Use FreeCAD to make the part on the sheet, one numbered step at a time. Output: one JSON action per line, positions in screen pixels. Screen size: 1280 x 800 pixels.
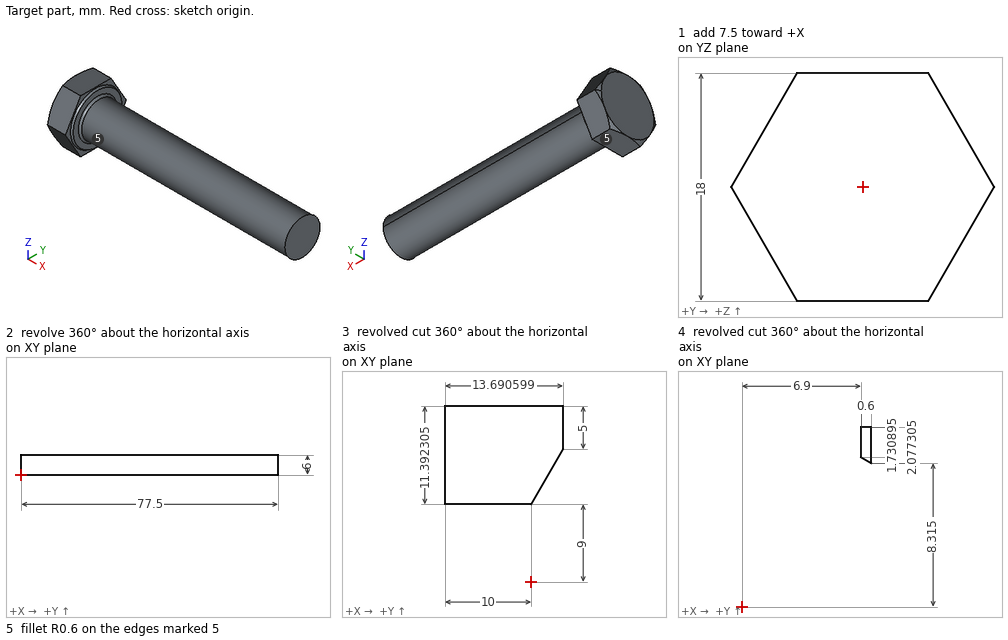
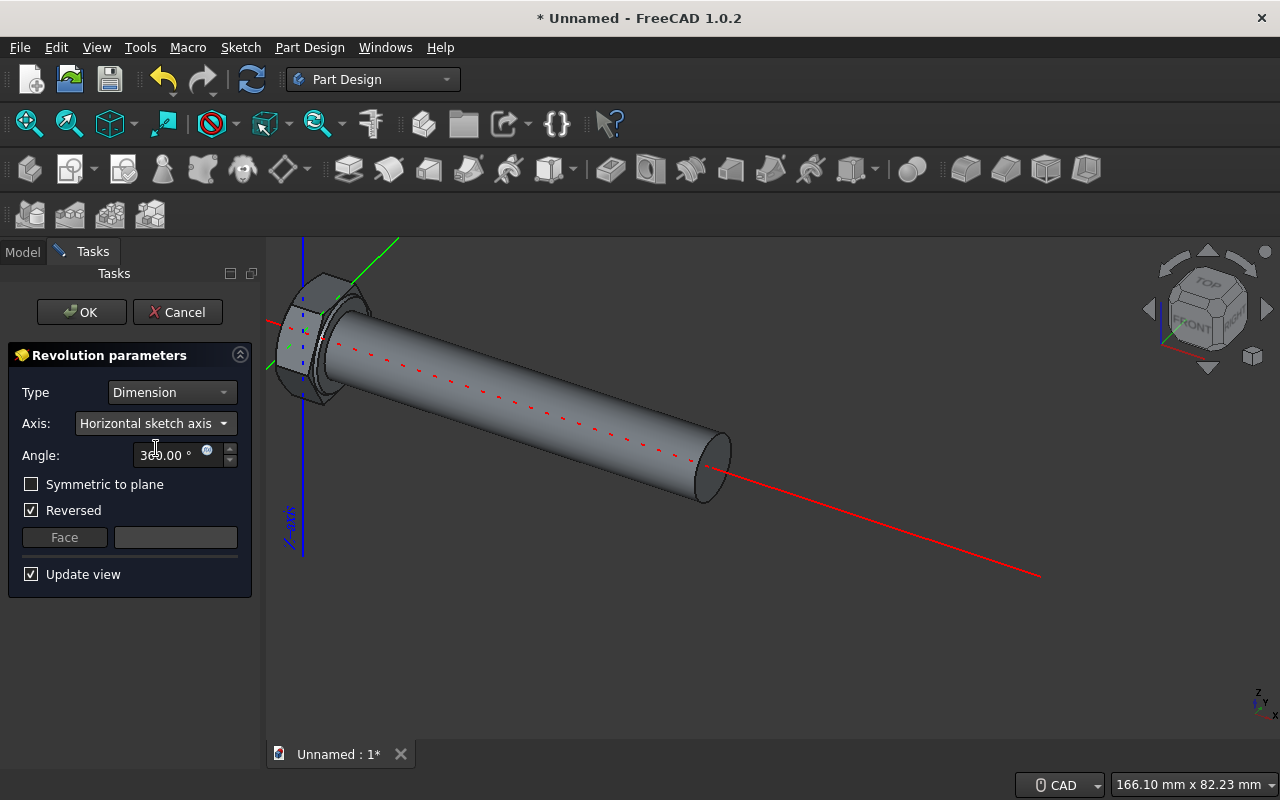
{"action": "left_click", "coordinate": [82, 312]}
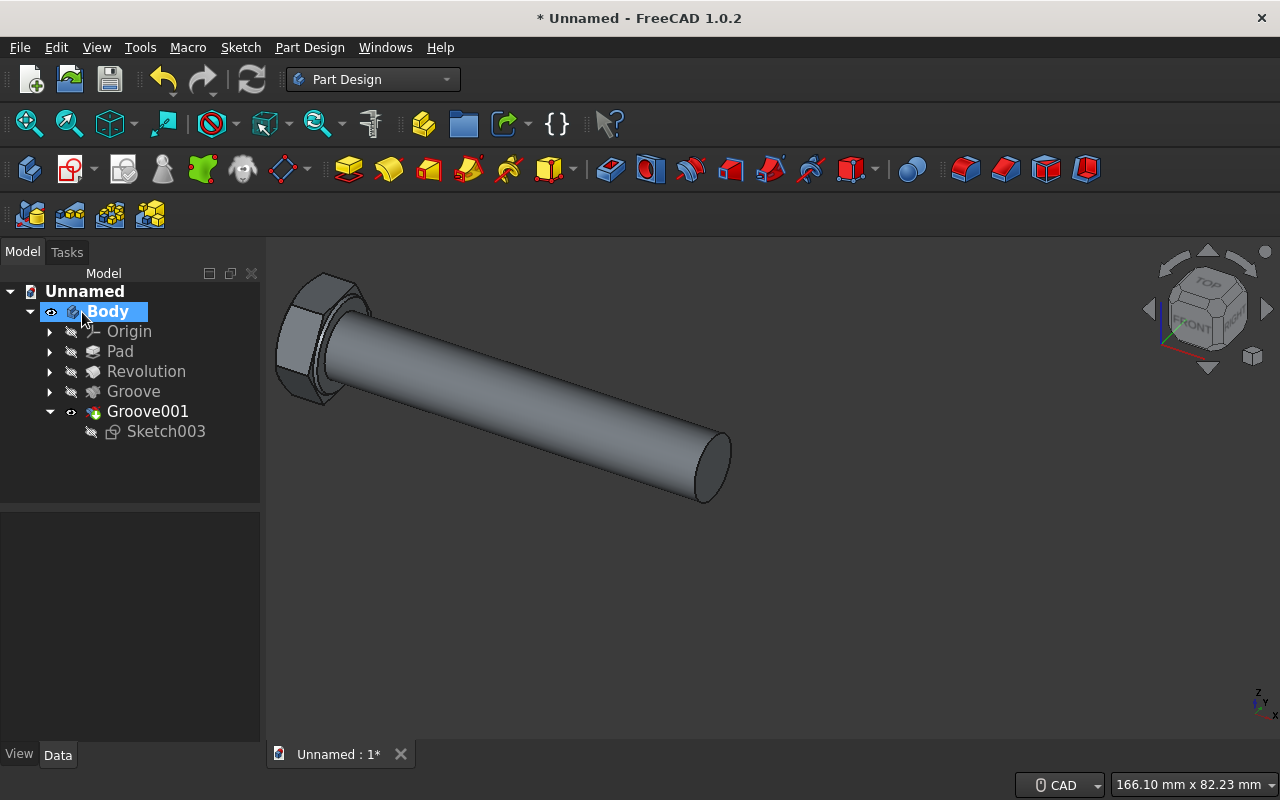
{"action": "key", "text": "0"}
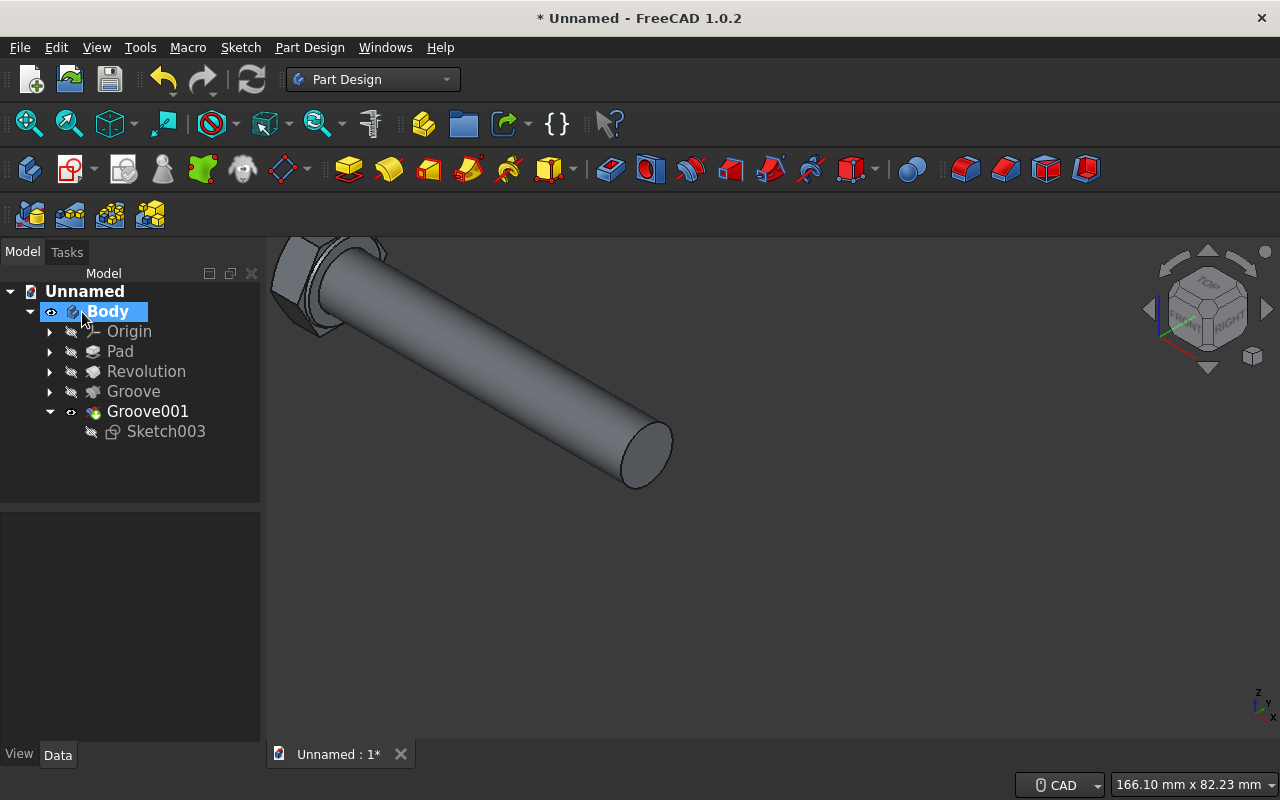
{"action": "left_click", "coordinate": [30, 124]}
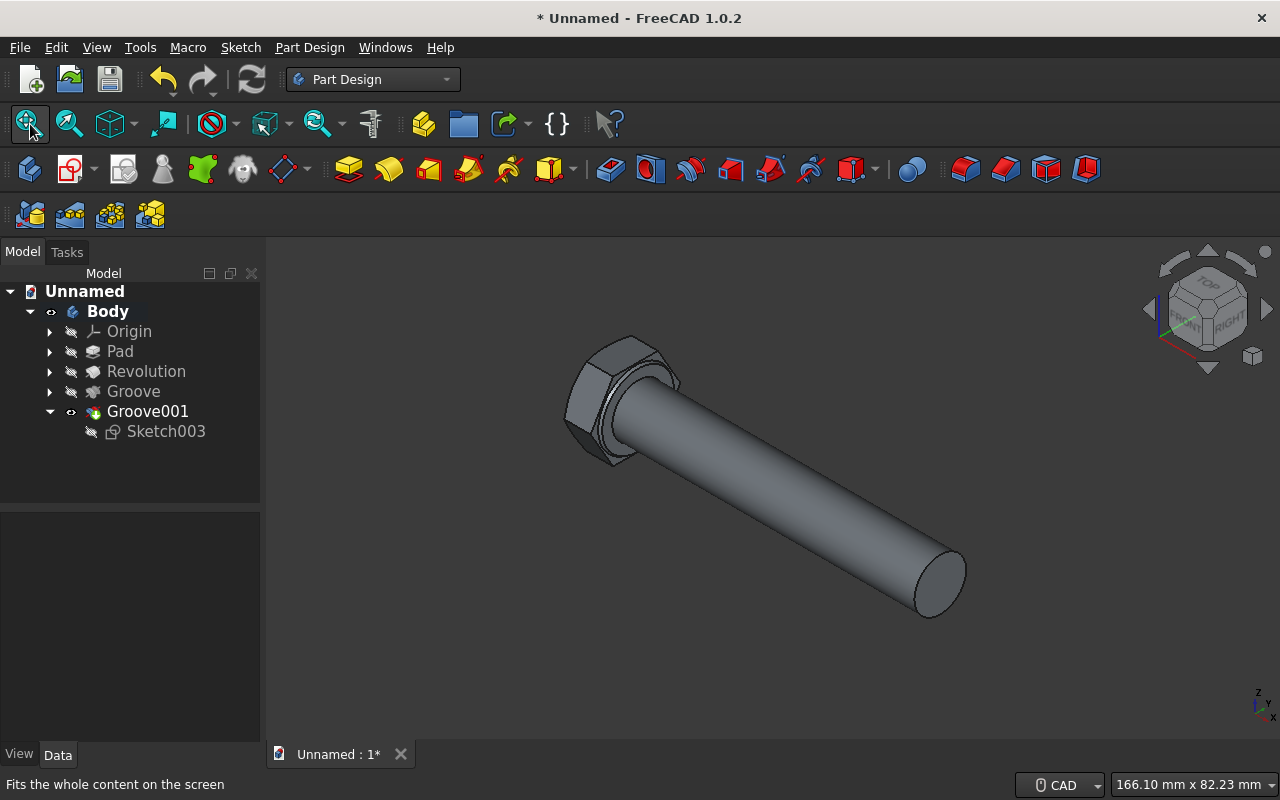
{"action": "key", "text": "2"}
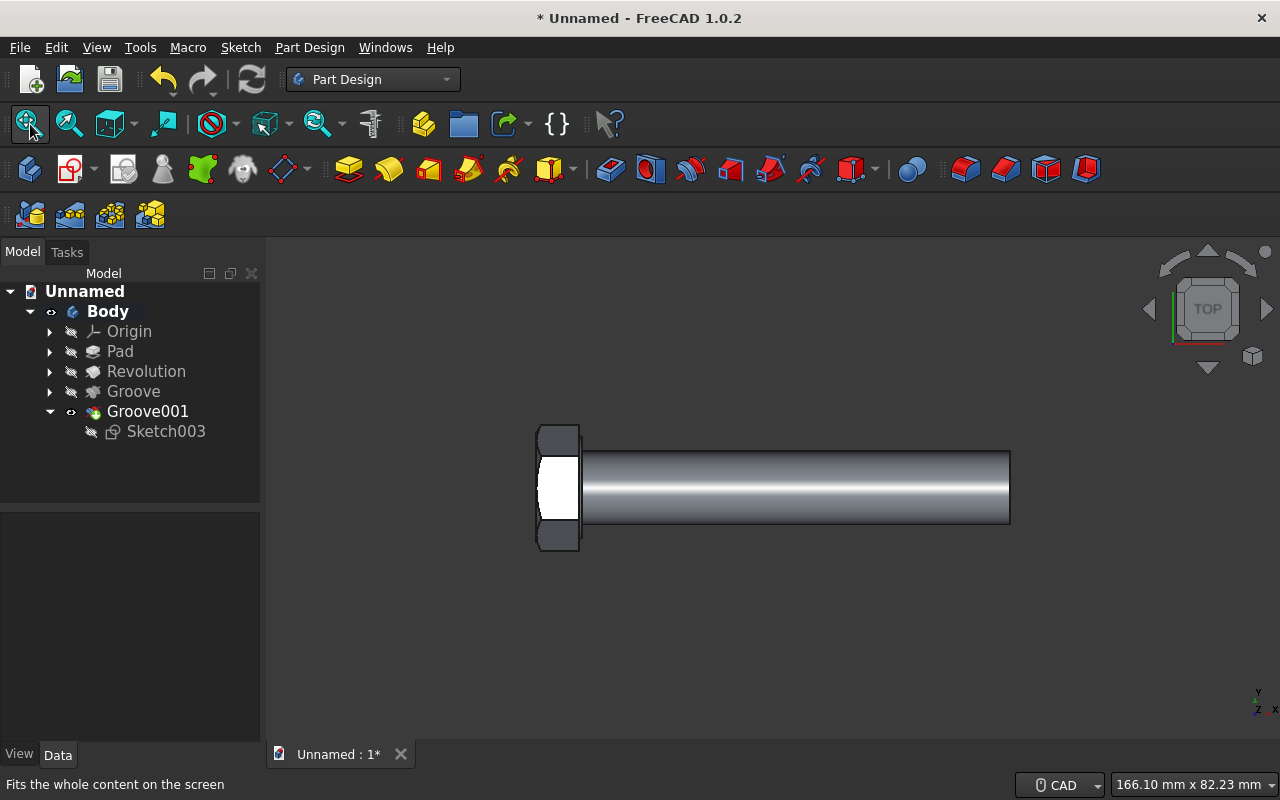
{"action": "key", "text": "1"}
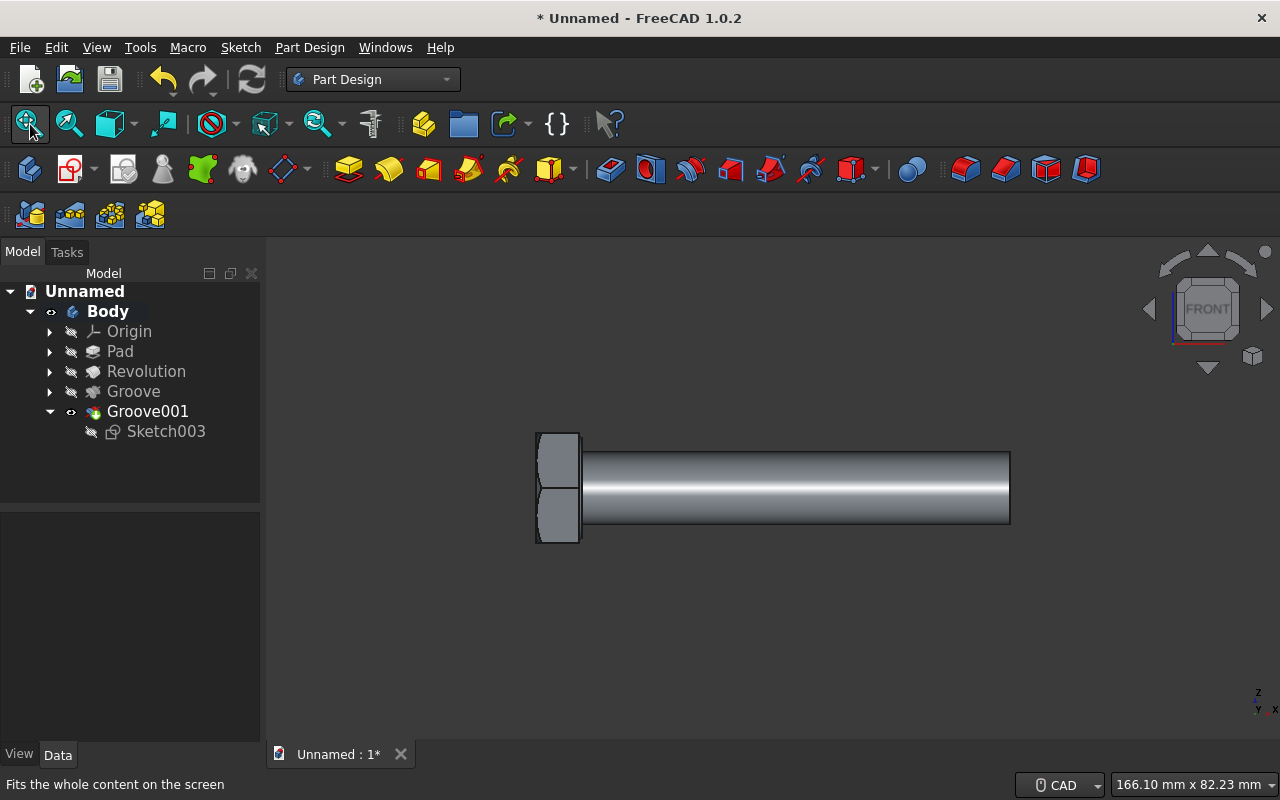
{"action": "key", "text": "3"}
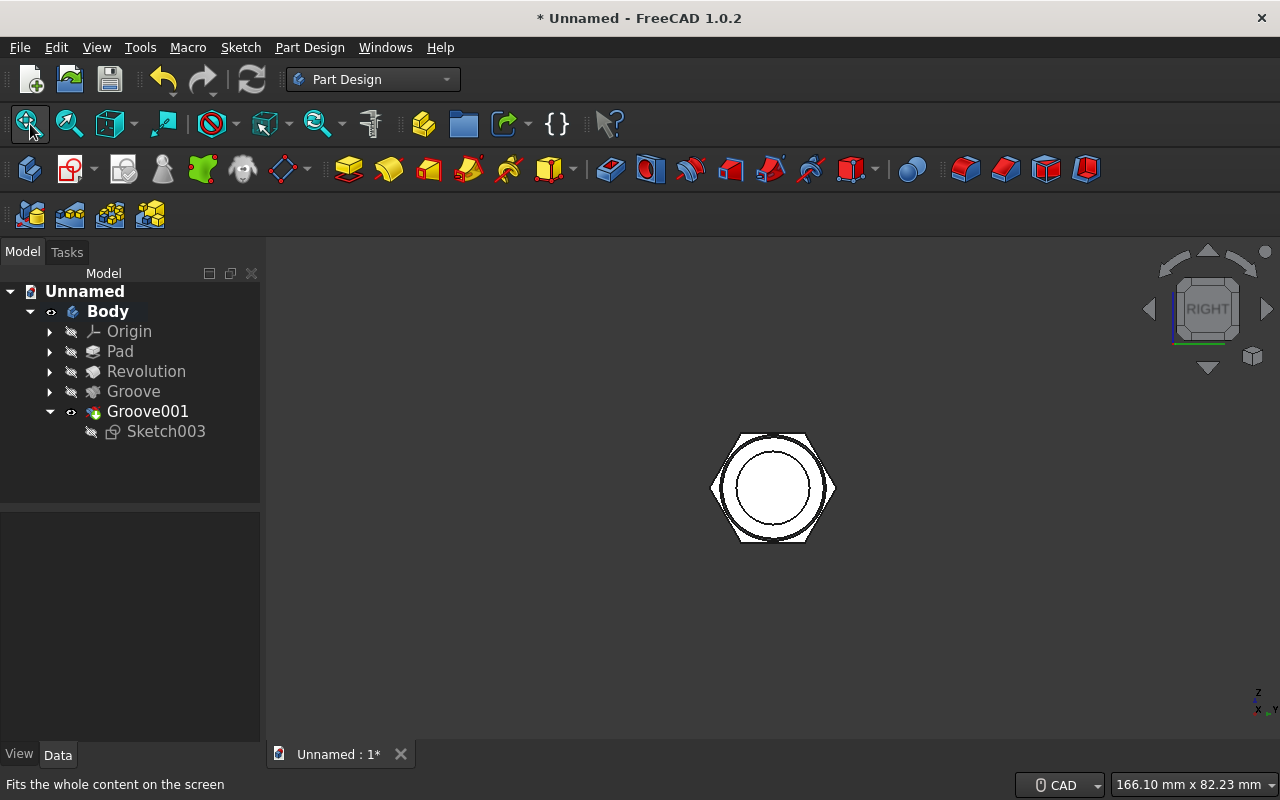
{"action": "left_click", "coordinate": [30, 124]}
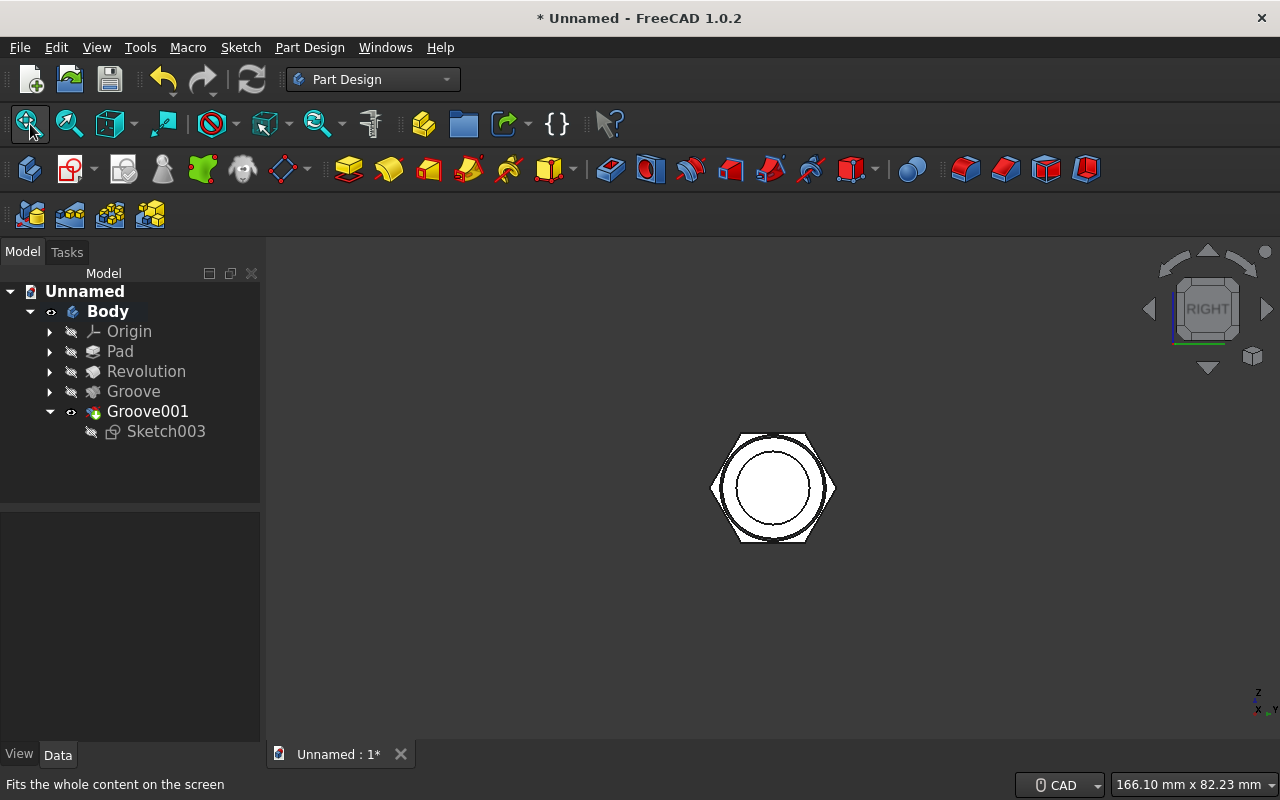
{"action": "key", "text": "5"}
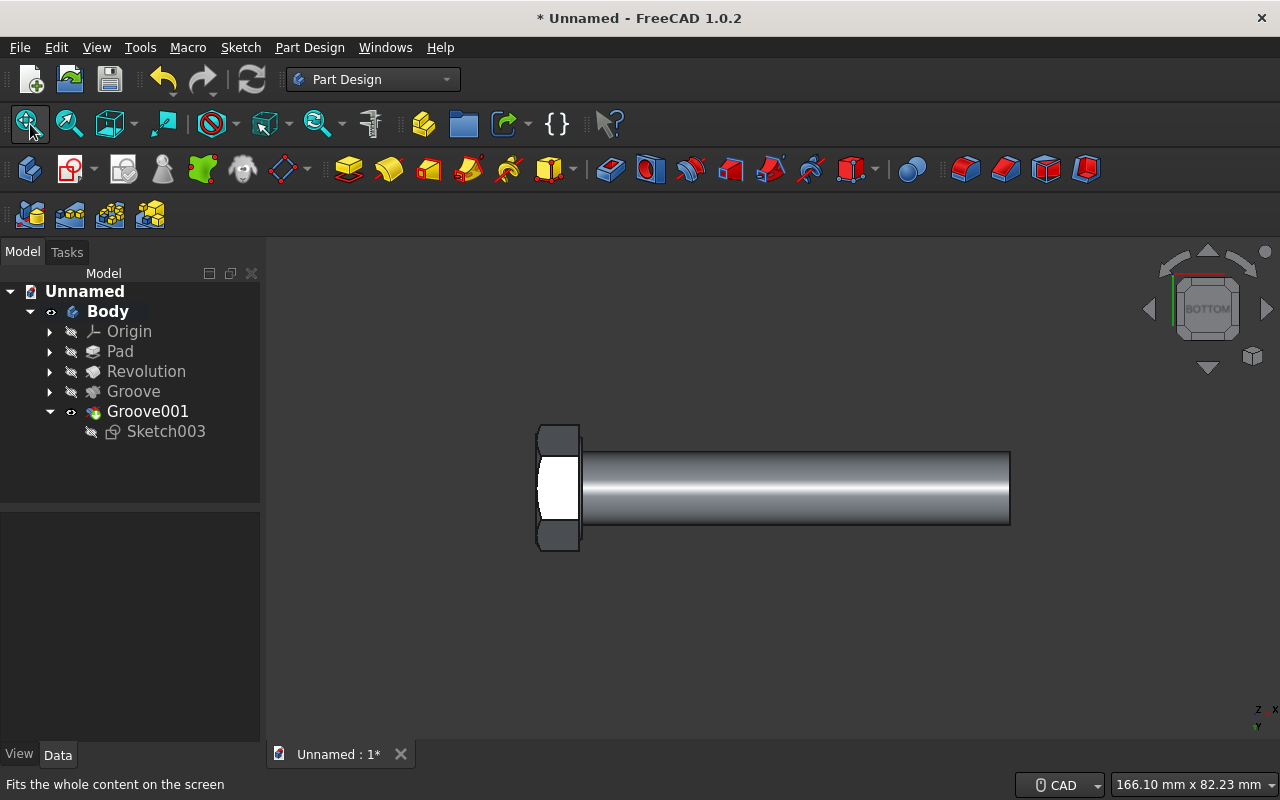
{"action": "key", "text": "4"}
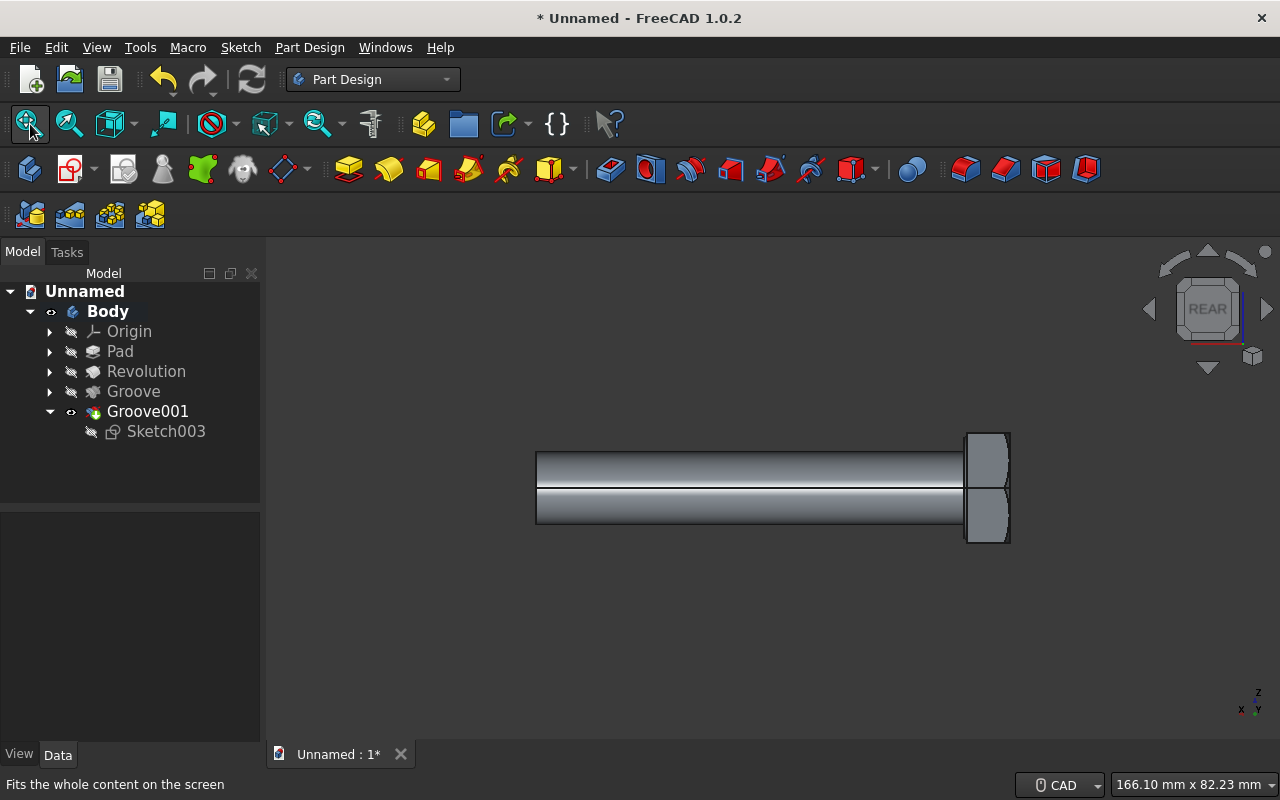
{"action": "key", "text": "6"}